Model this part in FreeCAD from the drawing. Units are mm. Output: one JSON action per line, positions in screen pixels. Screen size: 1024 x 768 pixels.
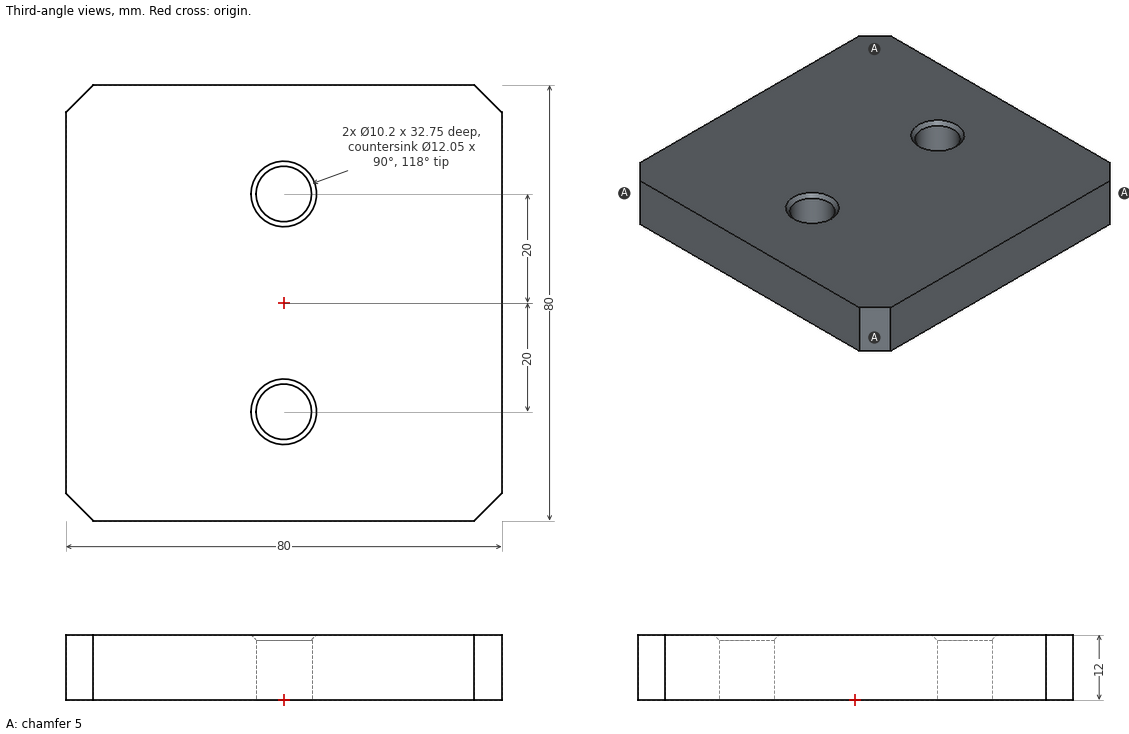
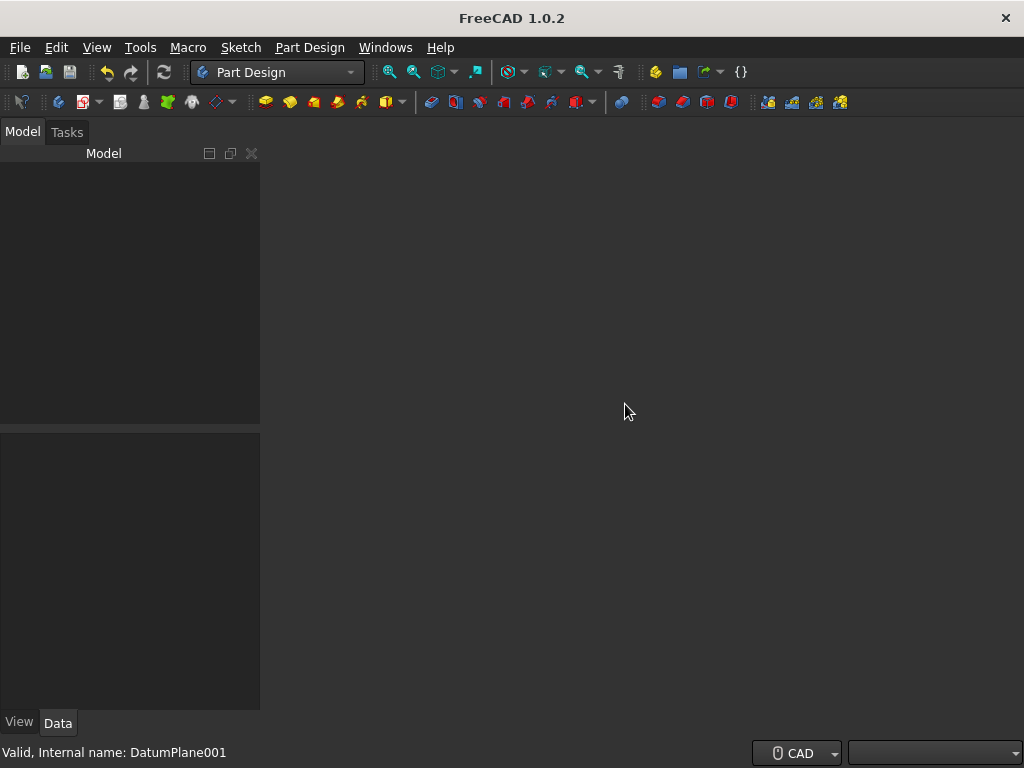
{"action": "key", "text": "ctrl+n"}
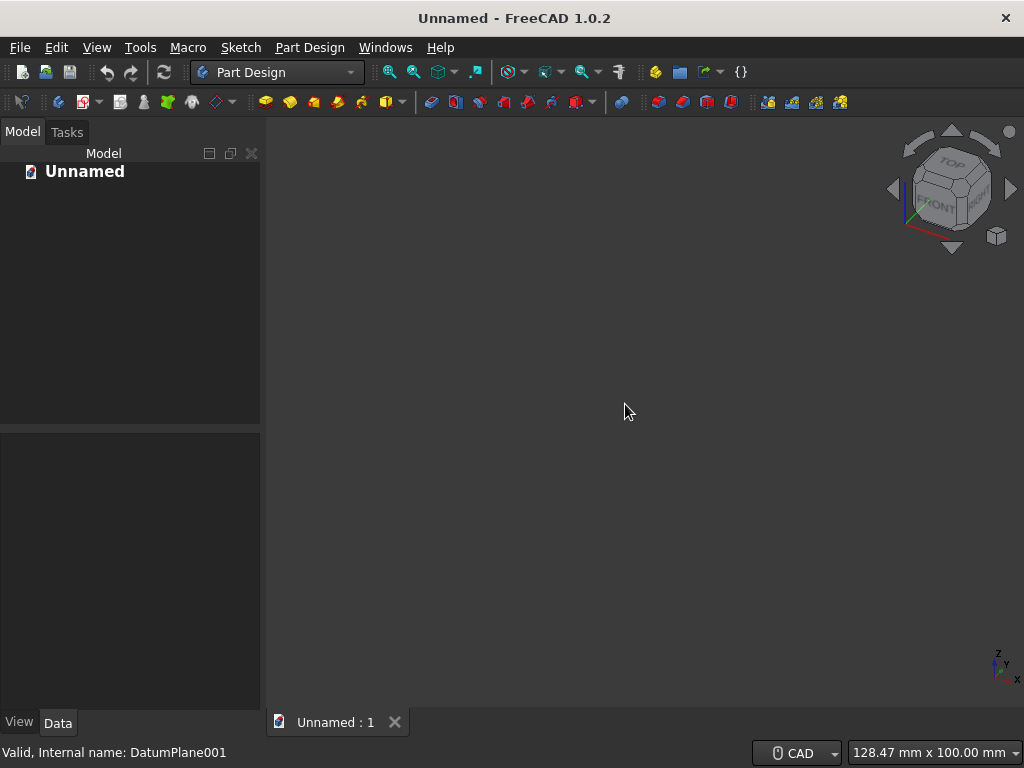
{"action": "left_click", "coordinate": [84, 102]}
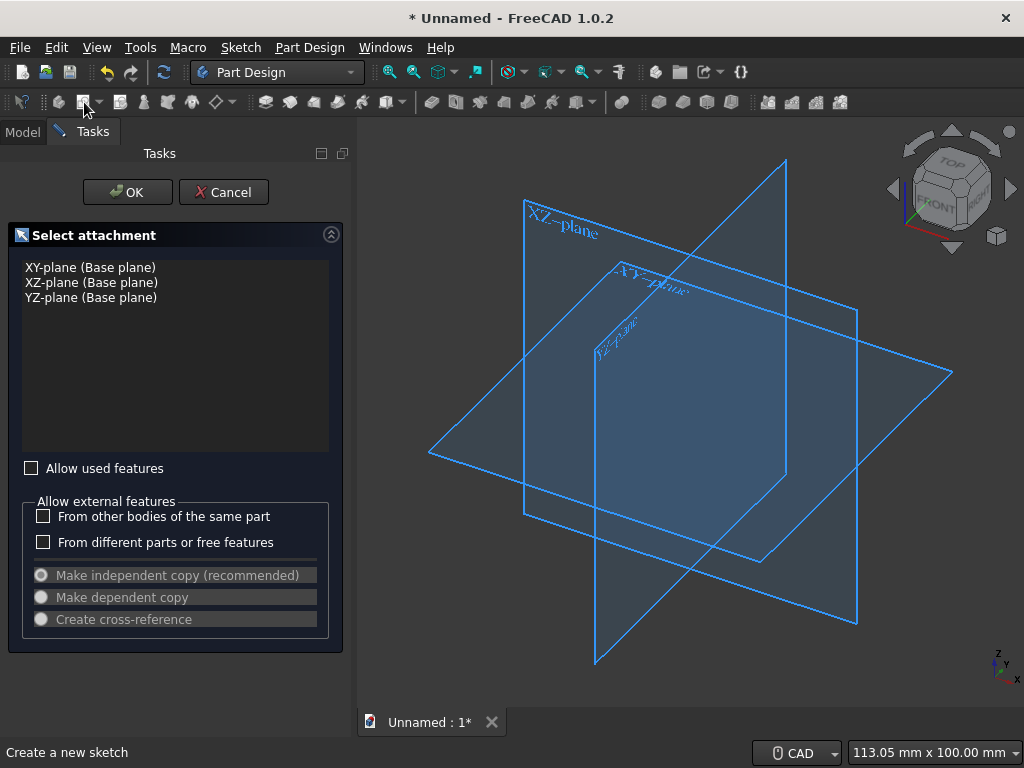
{"action": "left_click", "coordinate": [82, 268]}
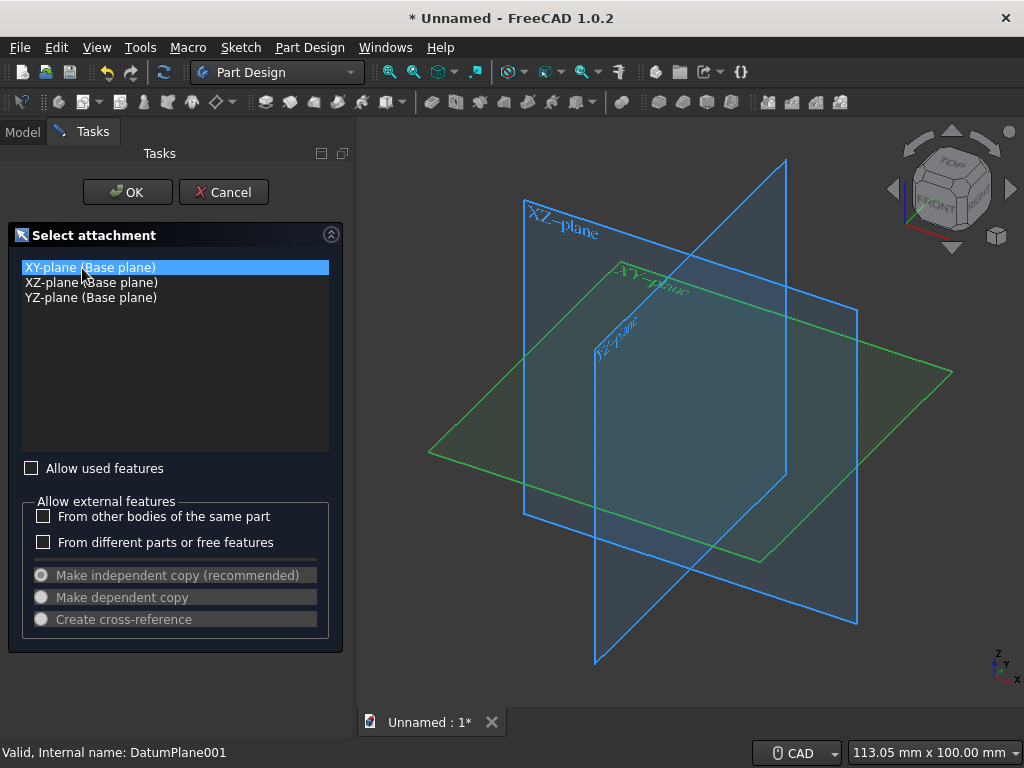
{"action": "left_click", "coordinate": [128, 192]}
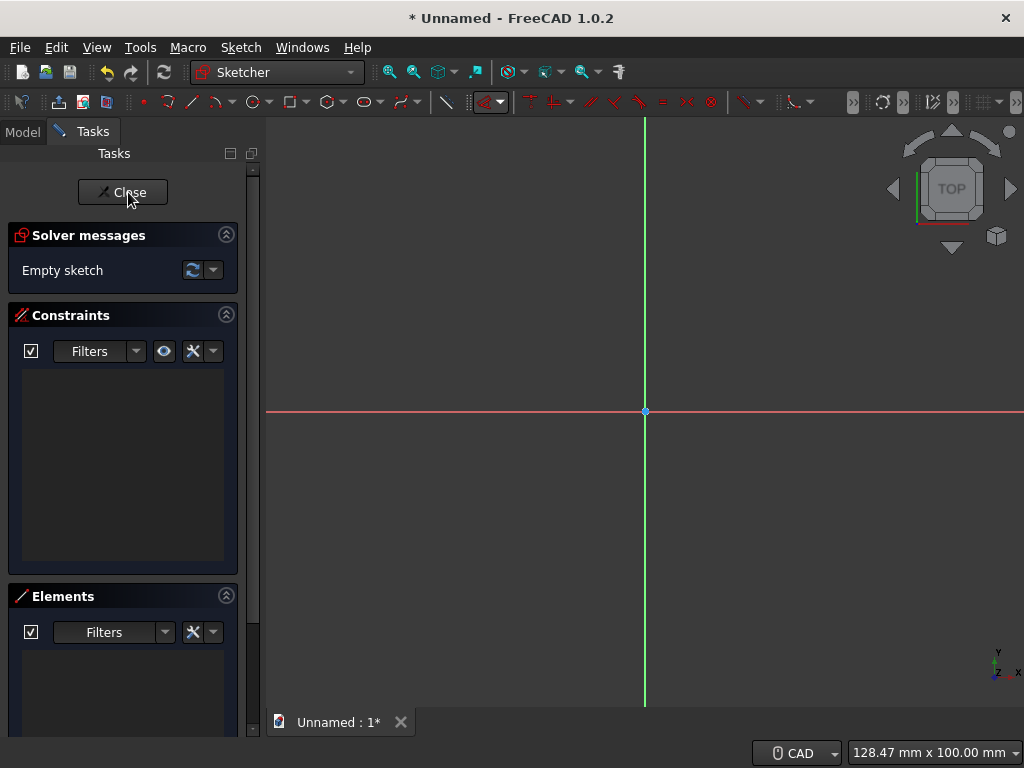
{"action": "scroll", "coordinate": [294, 412], "scroll_direction": "down", "scroll_amount": 1}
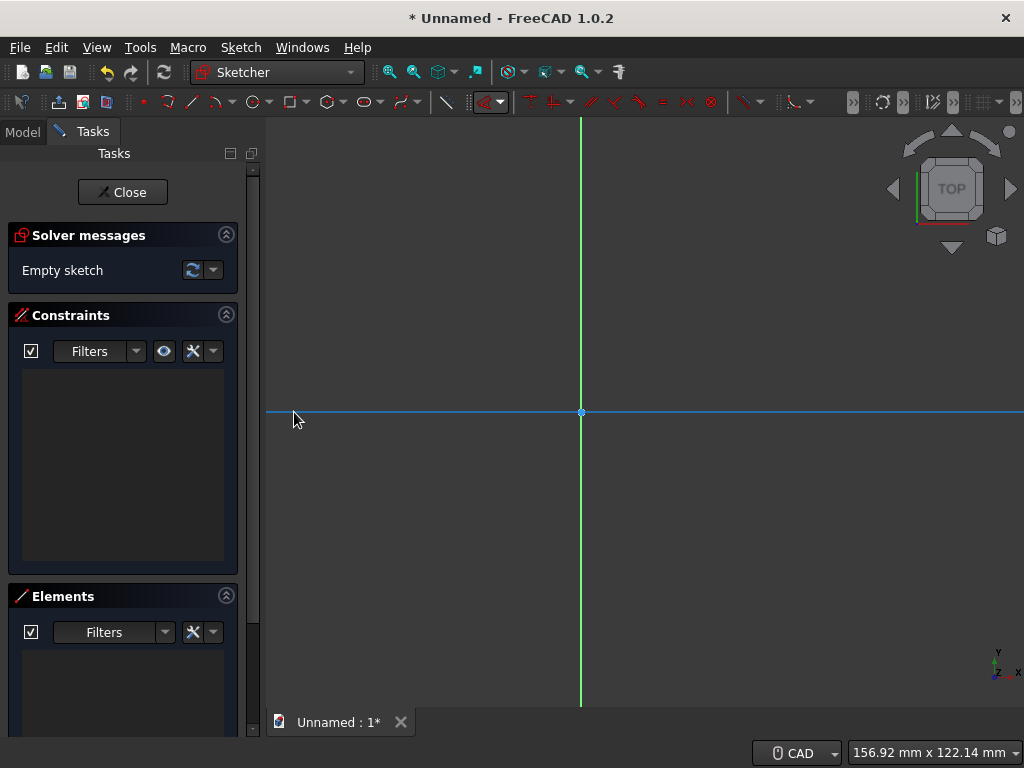
{"action": "key", "text": "g v"}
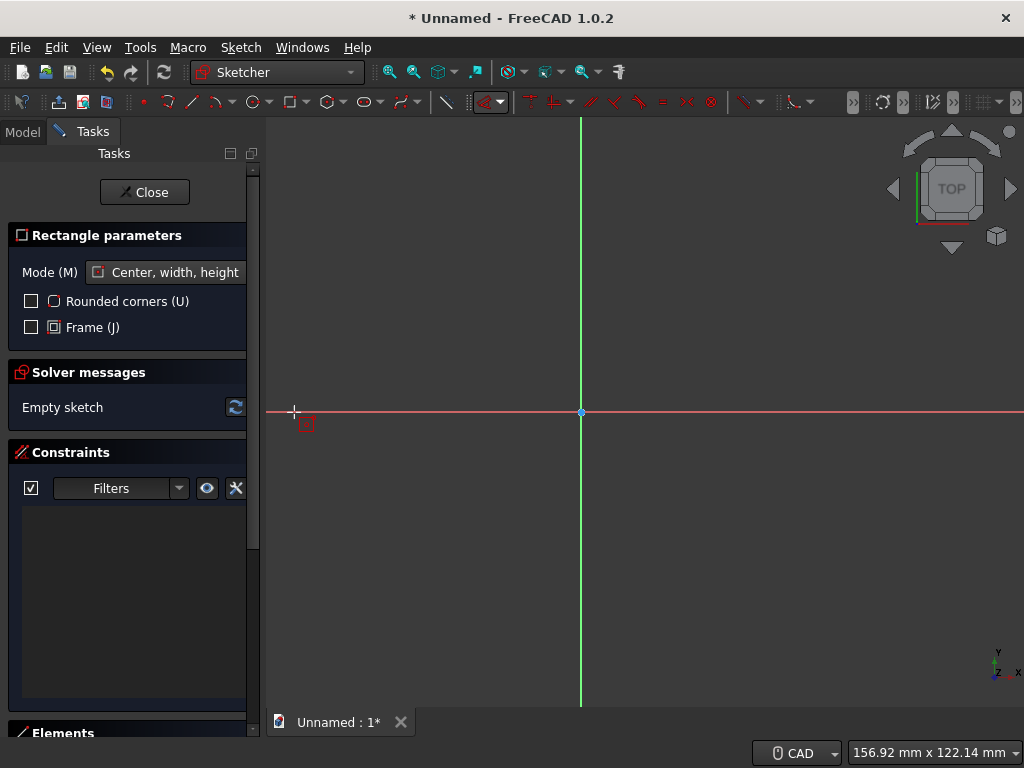
{"action": "left_click", "coordinate": [581, 412]}
{"action": "mouse_move", "coordinate": [775, 219]}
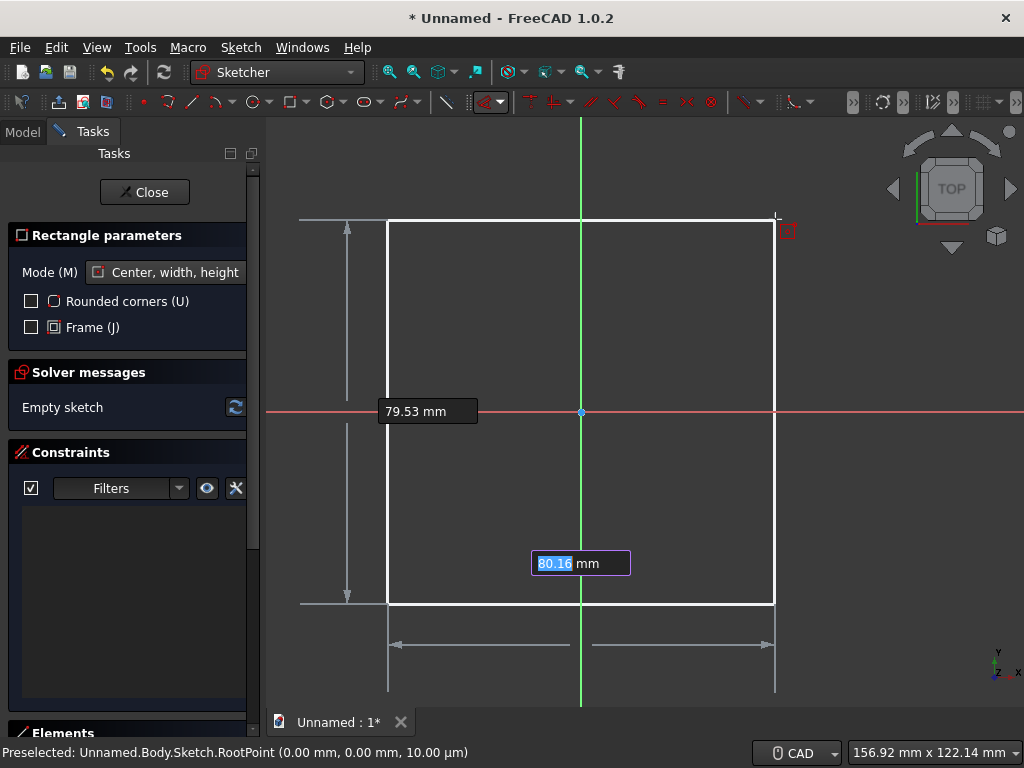
{"action": "type", "text": "80"}
{"action": "key", "text": "Tab"}
{"action": "type", "text": "80"}
{"action": "key", "text": "Return"}
{"action": "key", "text": "Escape"}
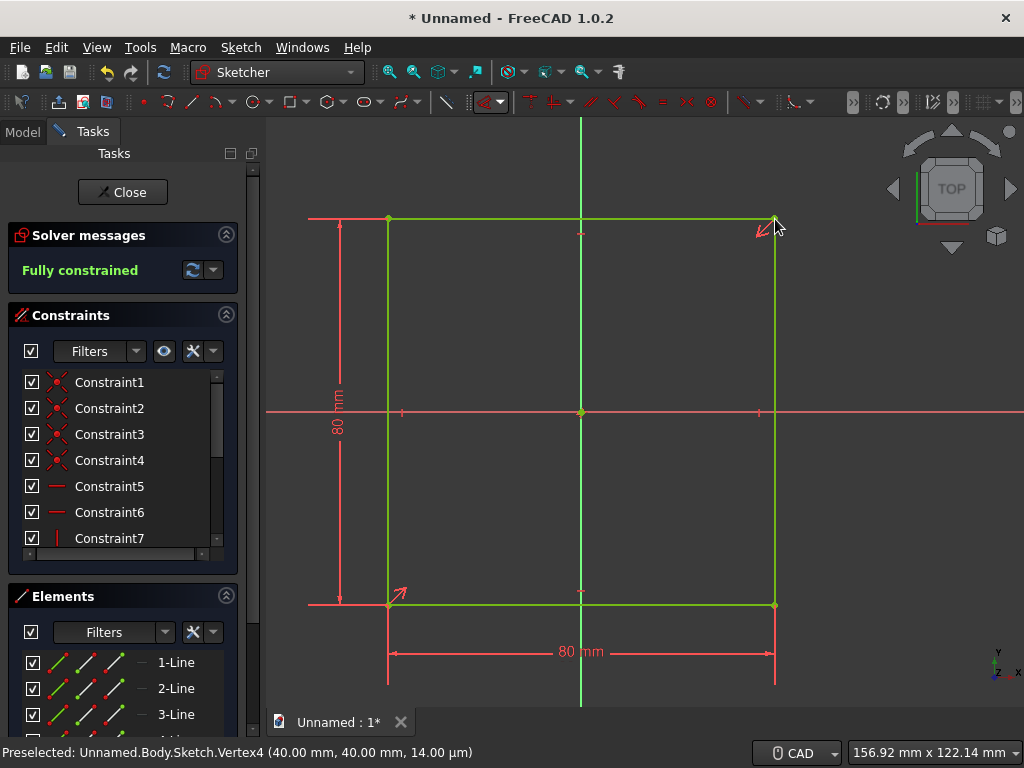
{"action": "left_click", "coordinate": [123, 192]}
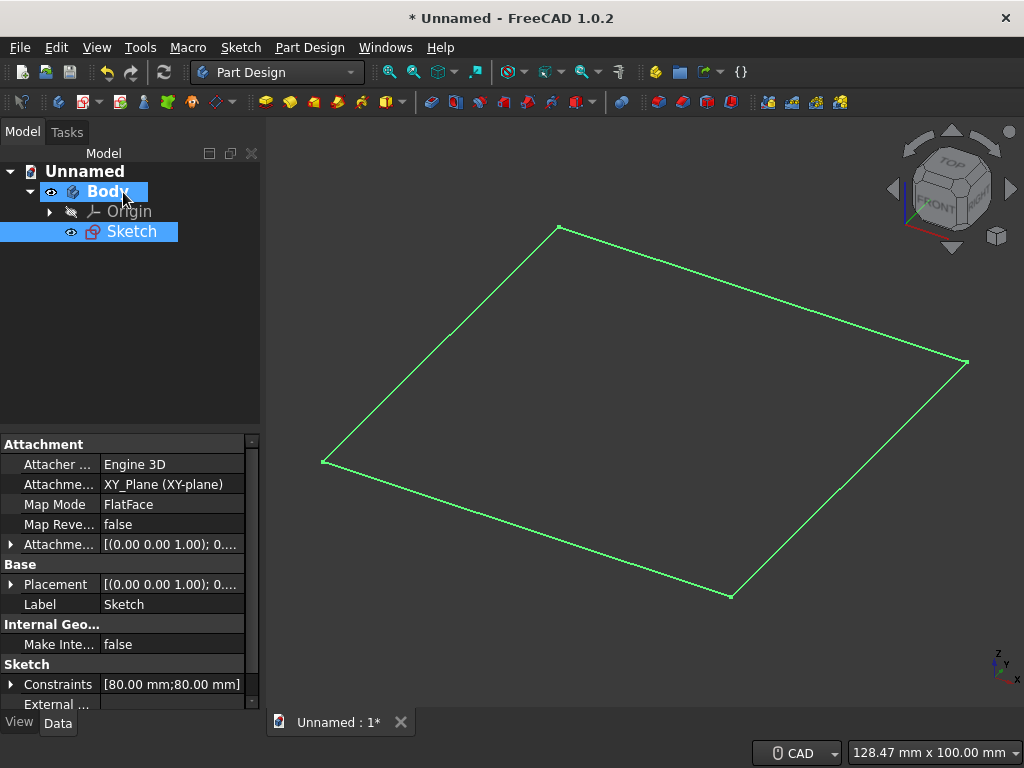
{"action": "left_click", "coordinate": [266, 102]}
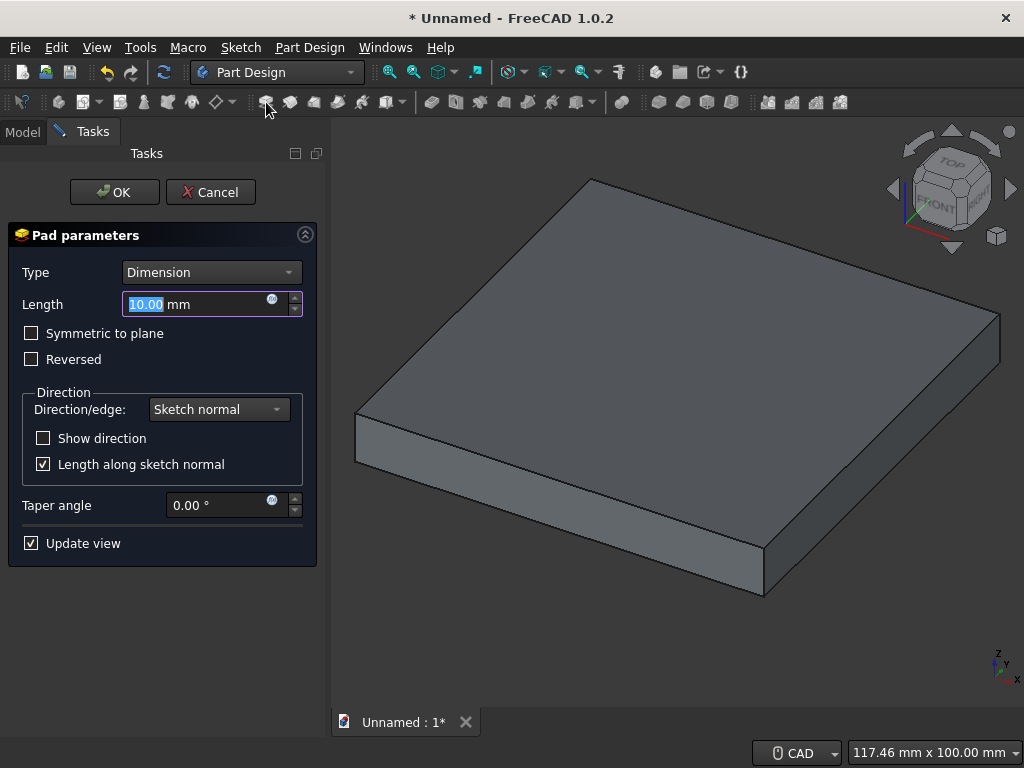
{"action": "type", "text": "12"}
{"action": "key", "text": "Tab"}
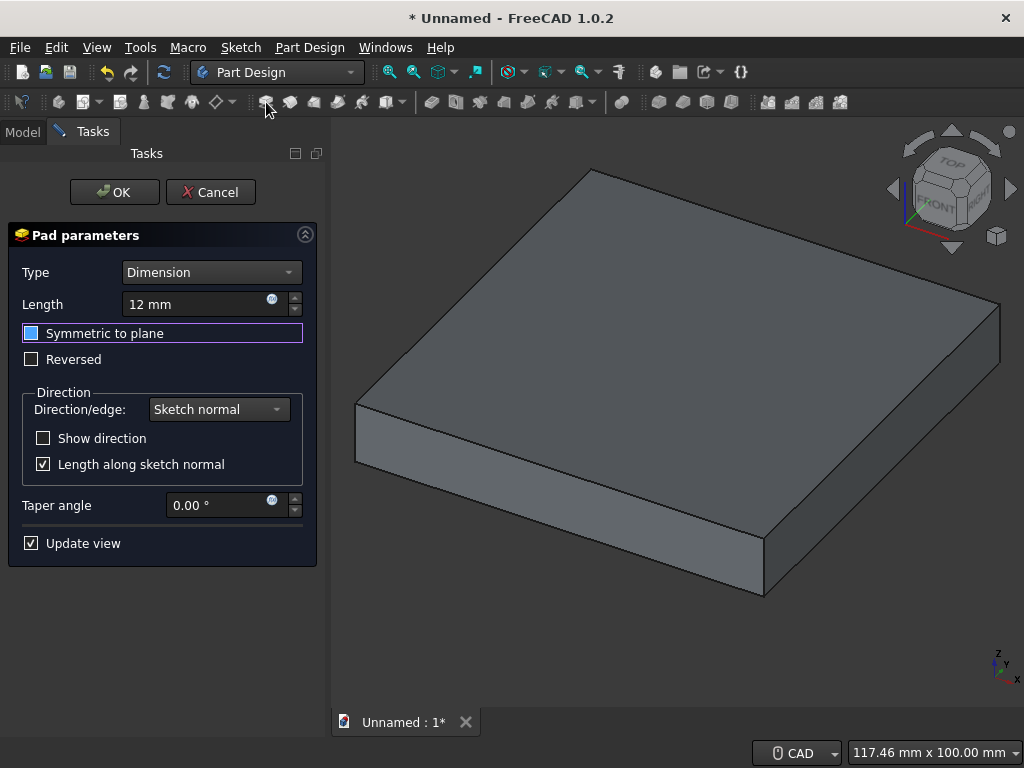
{"action": "left_click", "coordinate": [115, 192]}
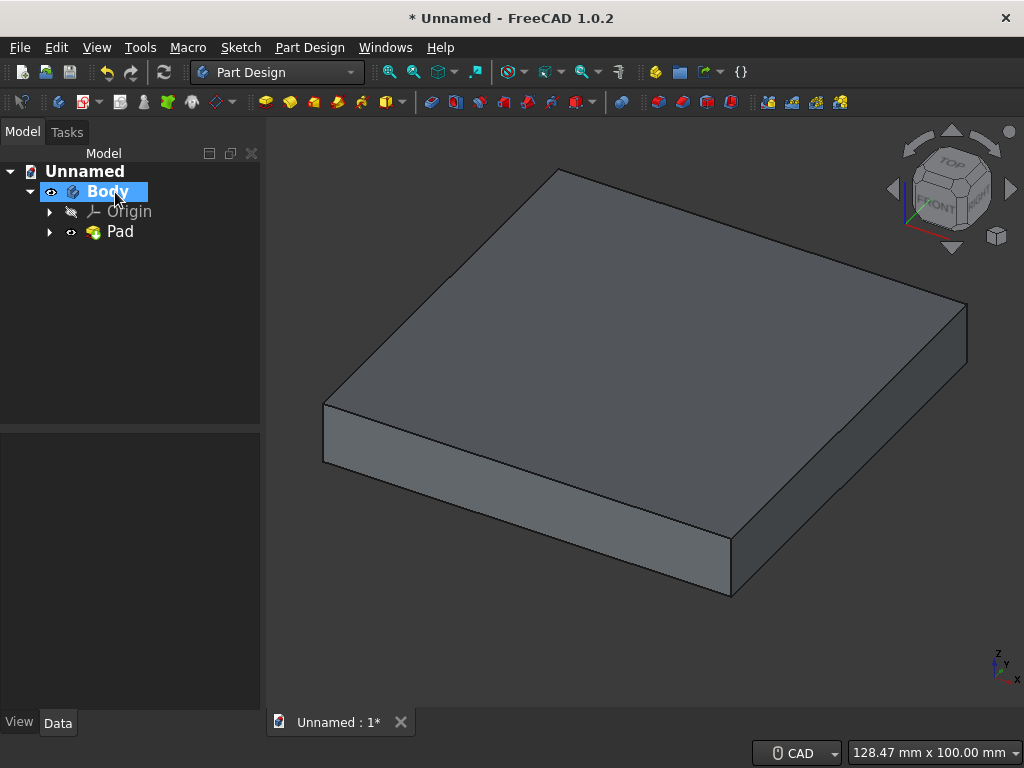
{"action": "left_click", "coordinate": [731, 567]}